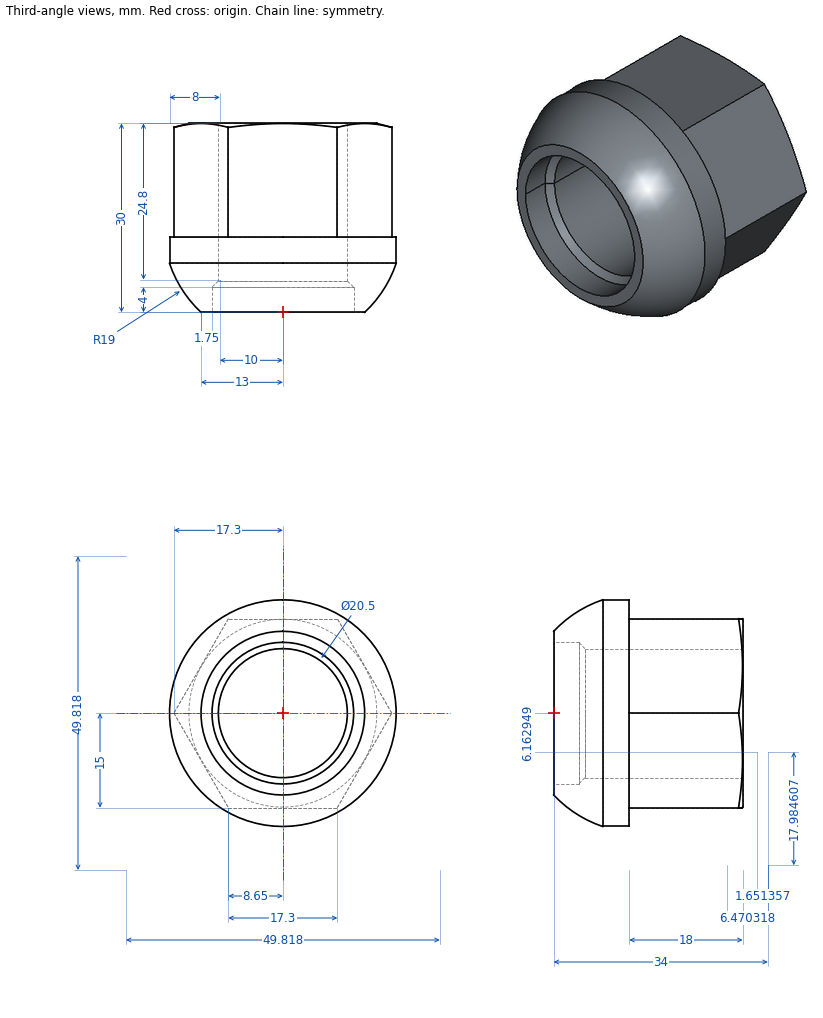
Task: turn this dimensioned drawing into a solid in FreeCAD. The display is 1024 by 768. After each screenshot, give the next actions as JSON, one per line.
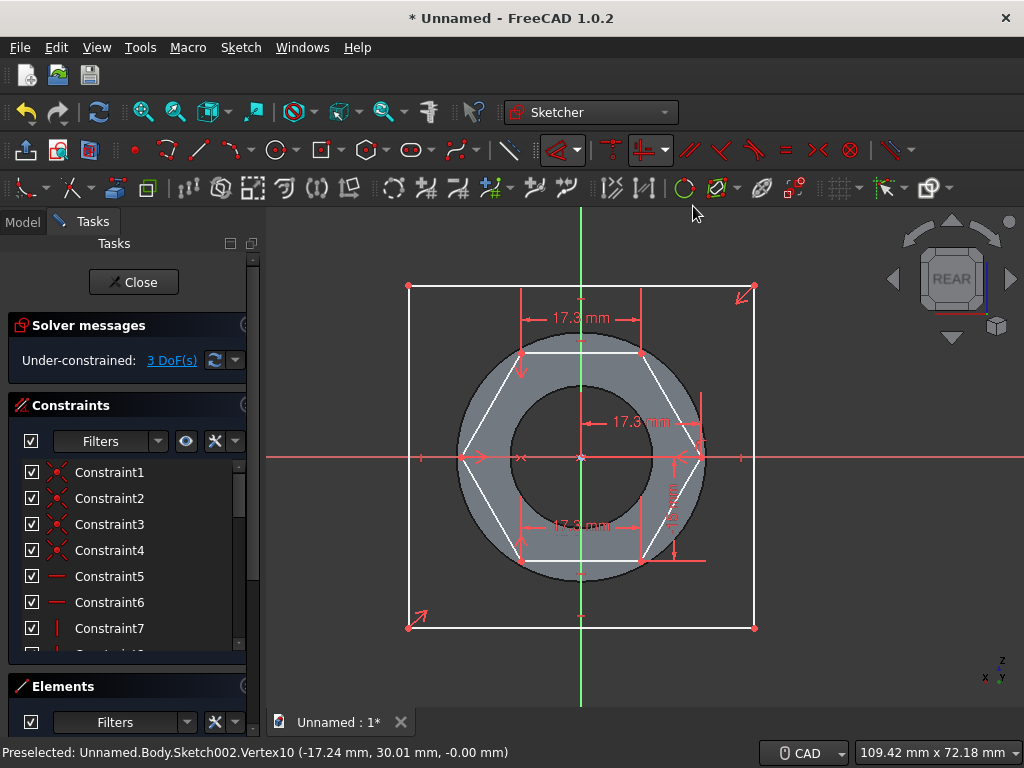
{"action": "left_click", "coordinate": [641, 561]}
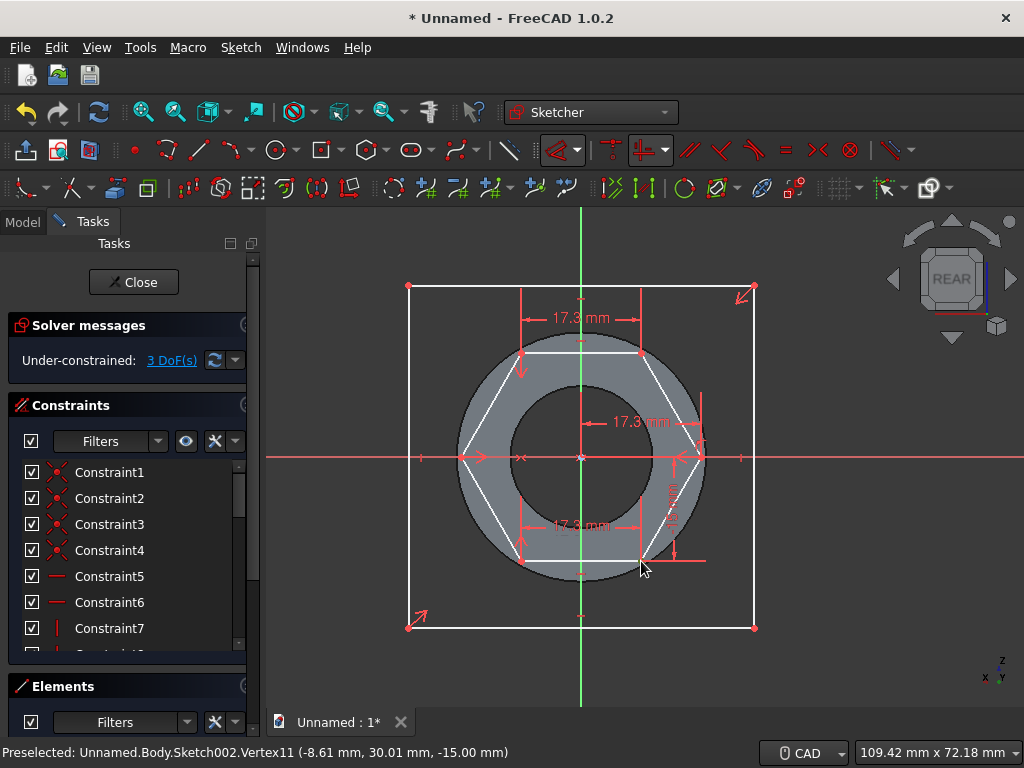
{"action": "key", "text": "l"}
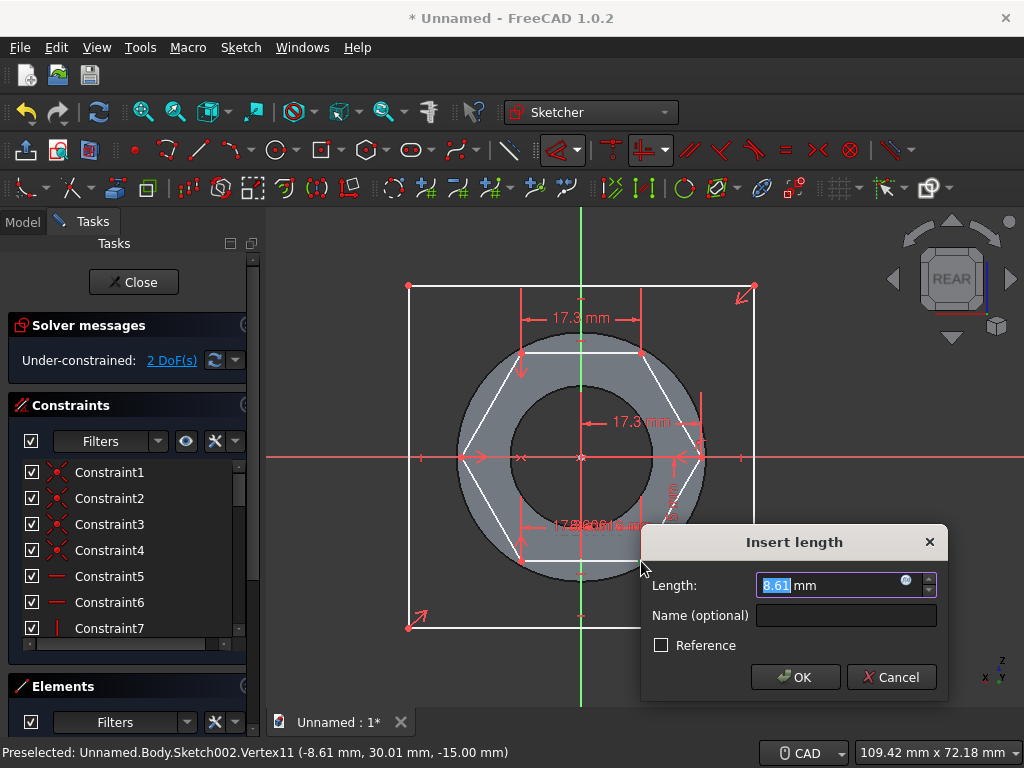
{"action": "type", "text": "8.65"}
{"action": "key", "text": "Return"}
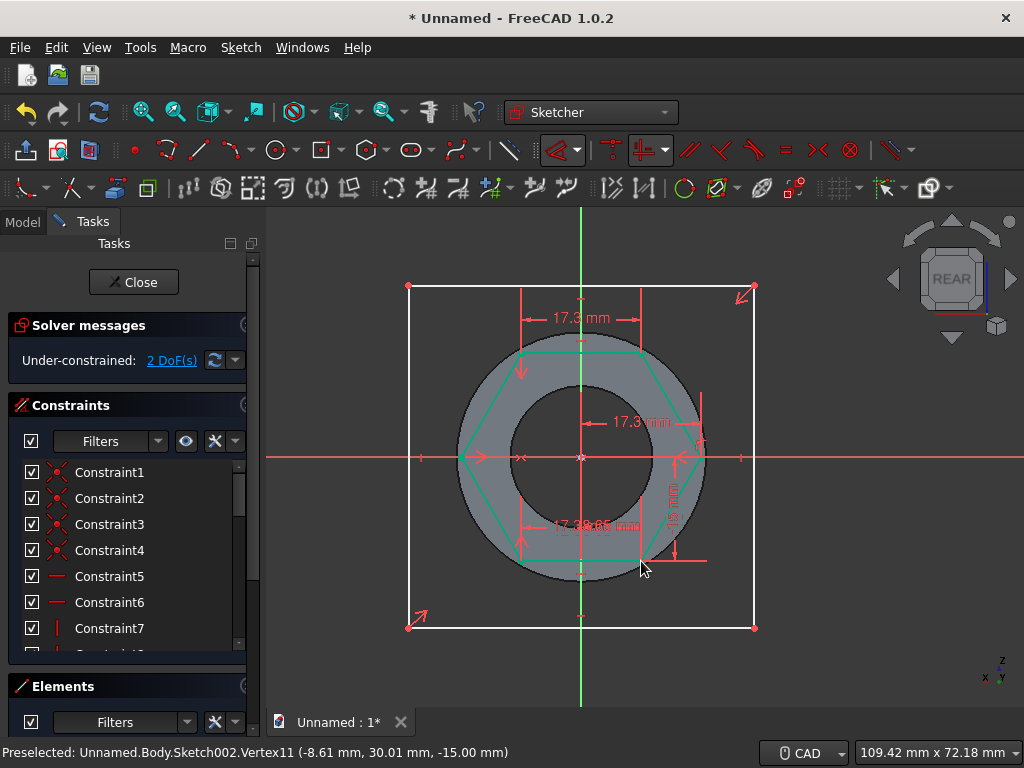
{"action": "left_click", "coordinate": [512, 628]}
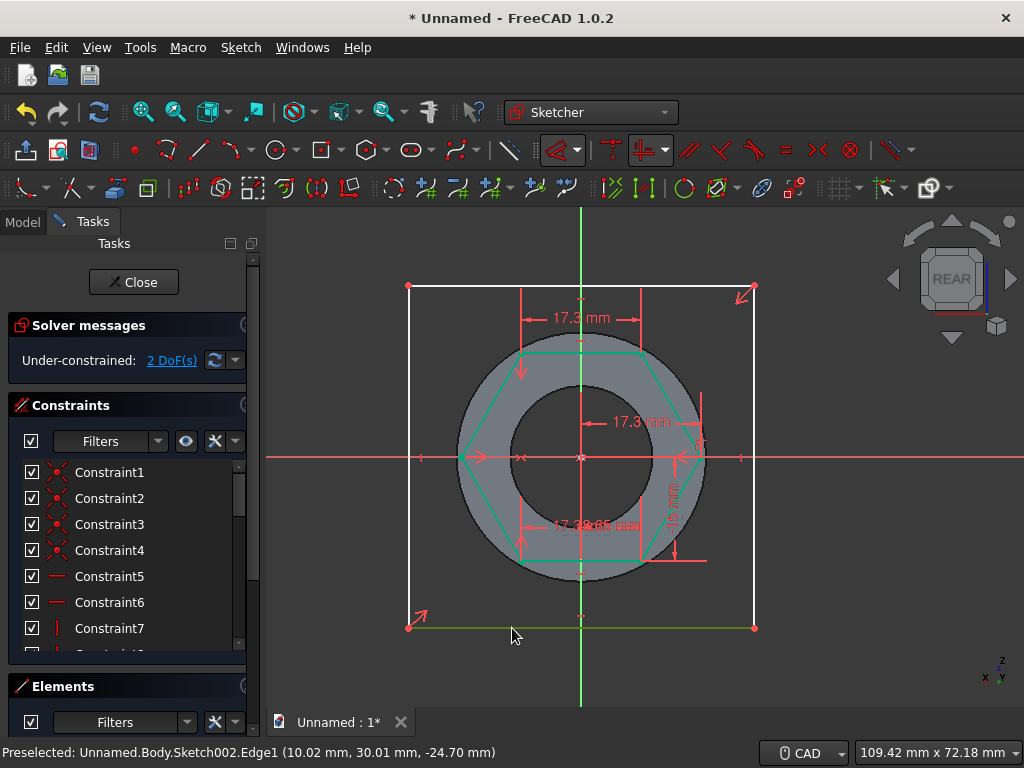
{"action": "key", "text": "l"}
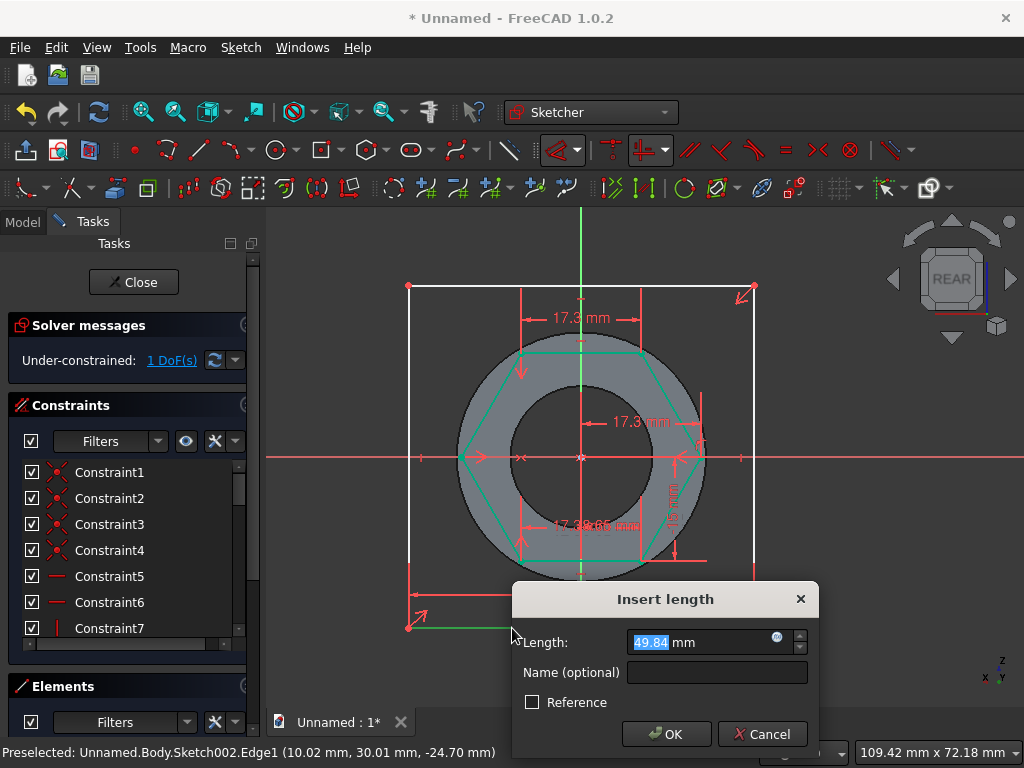
{"action": "type", "text": "49.818"}
{"action": "key", "text": "Return"}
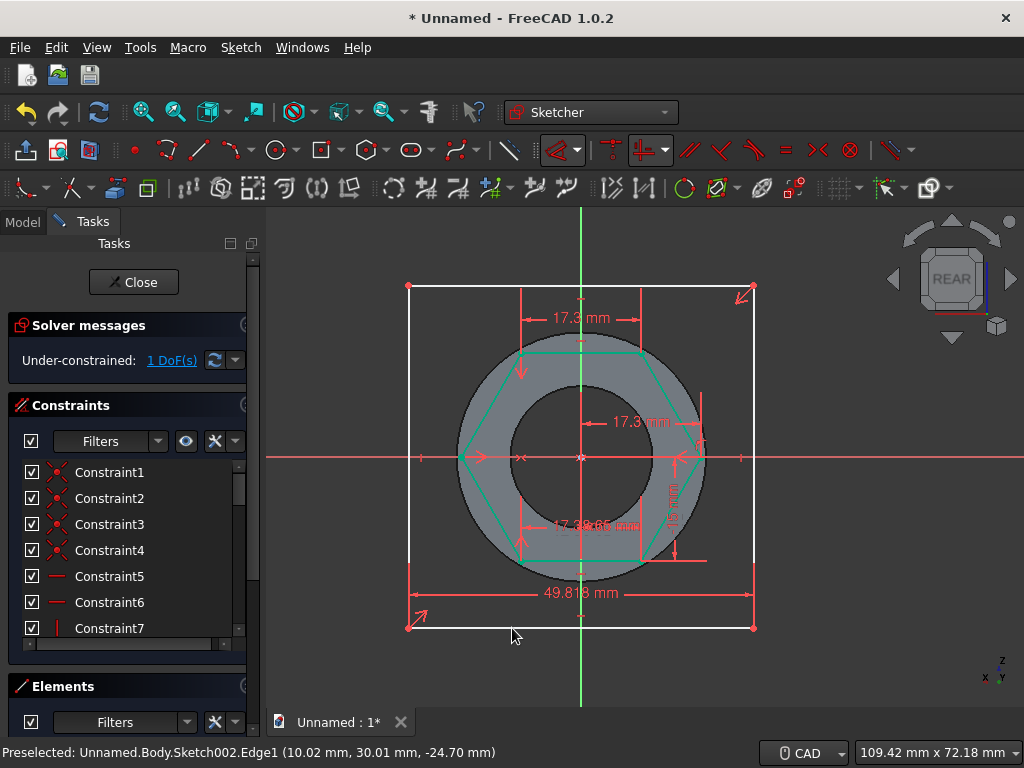
{"action": "left_click", "coordinate": [754, 526]}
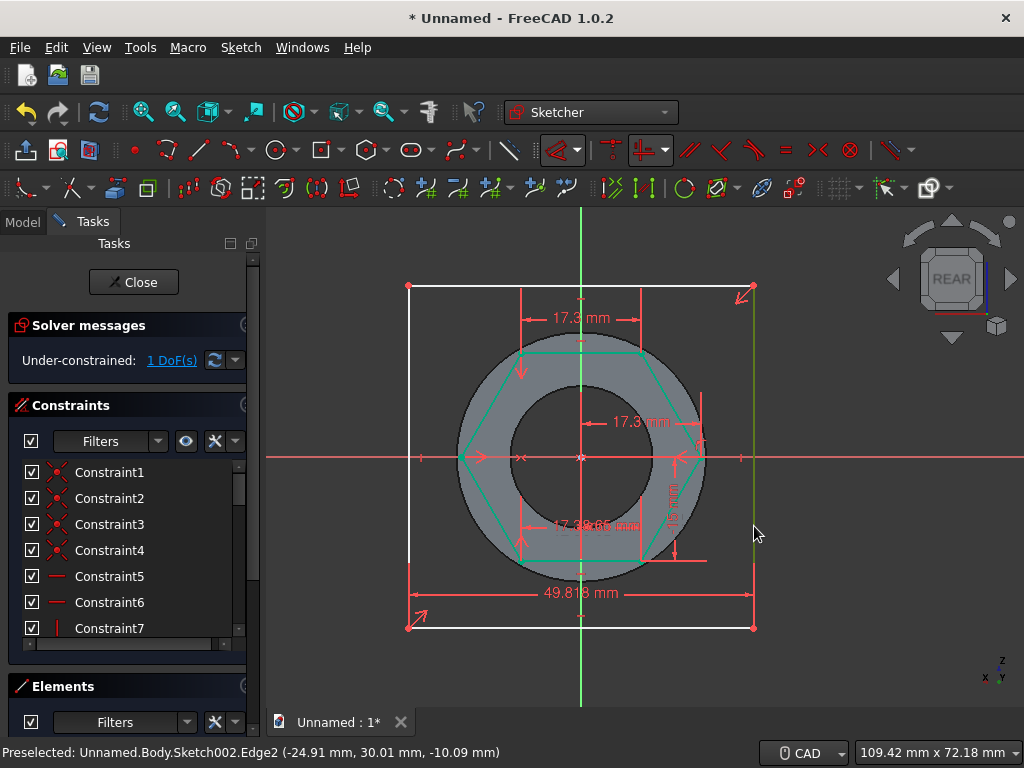
{"action": "key", "text": "i"}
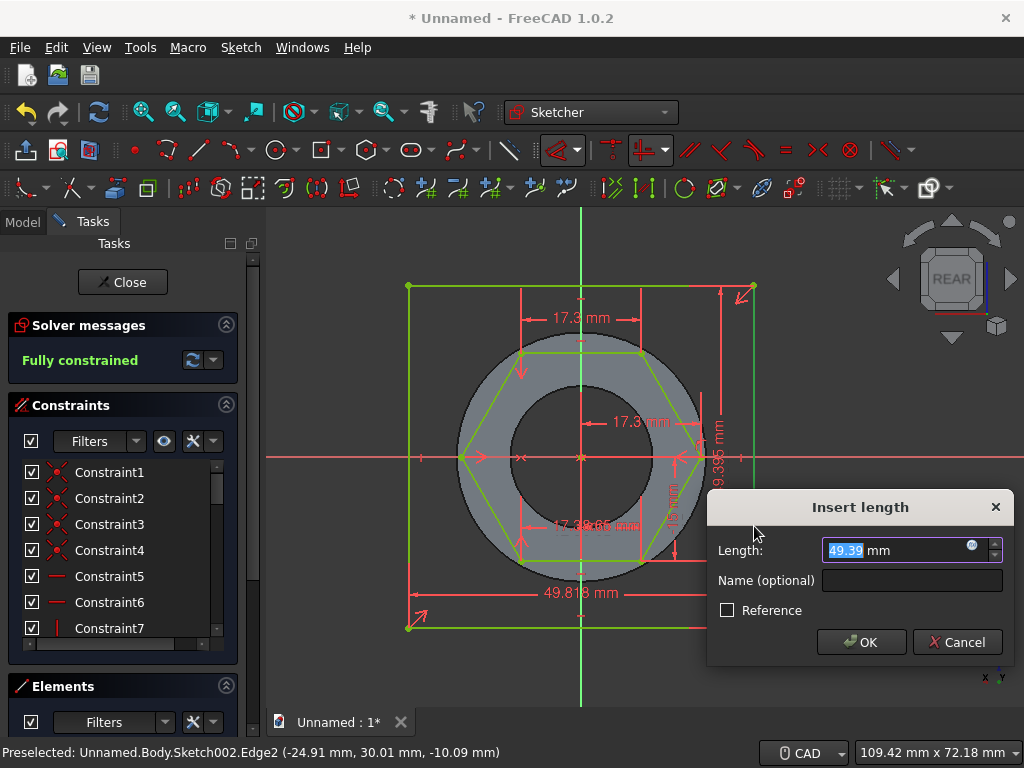
{"action": "type", "text": "49.818"}
{"action": "key", "text": "Return"}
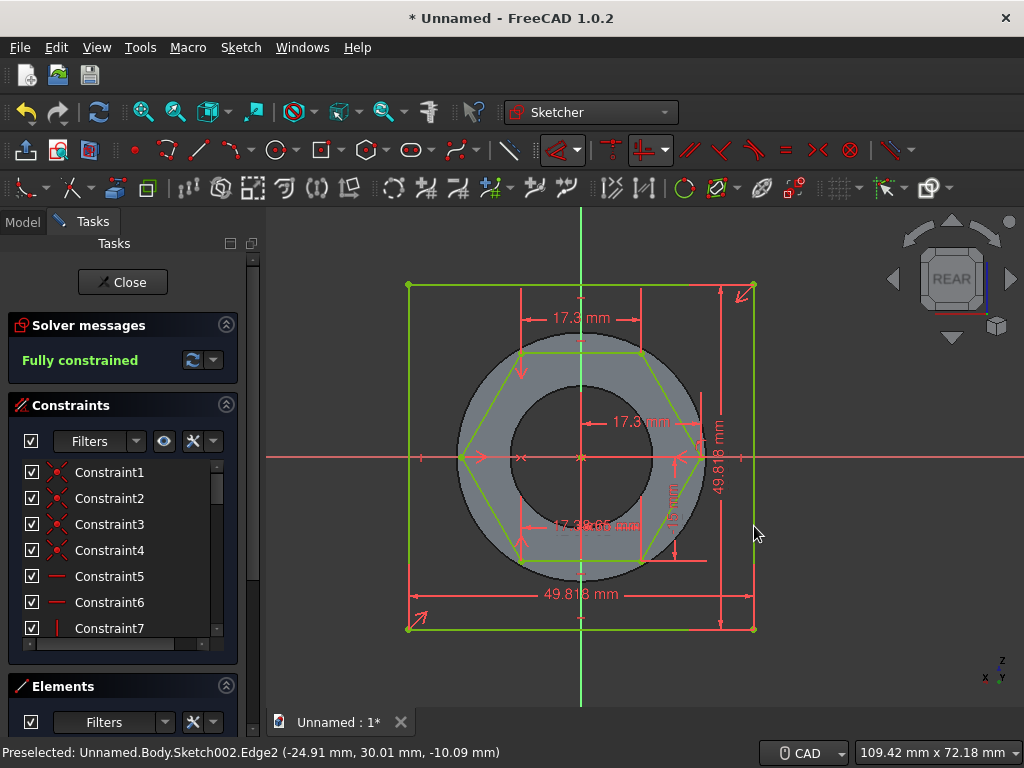
{"action": "left_click", "coordinate": [123, 282]}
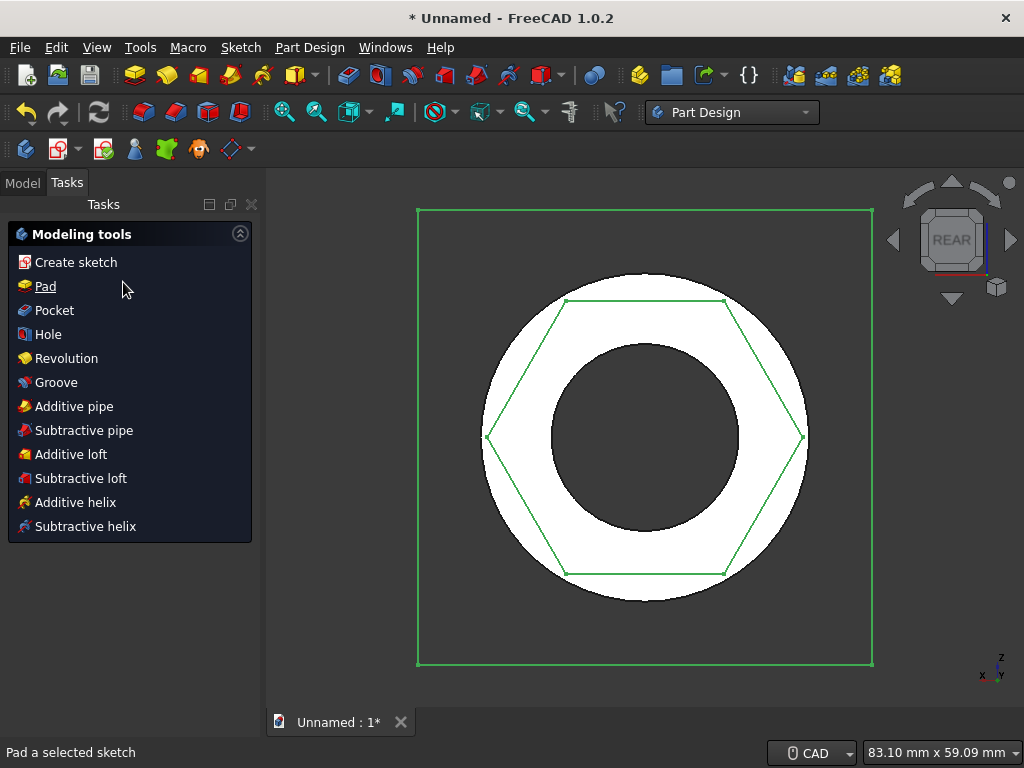
{"action": "left_click", "coordinate": [350, 76]}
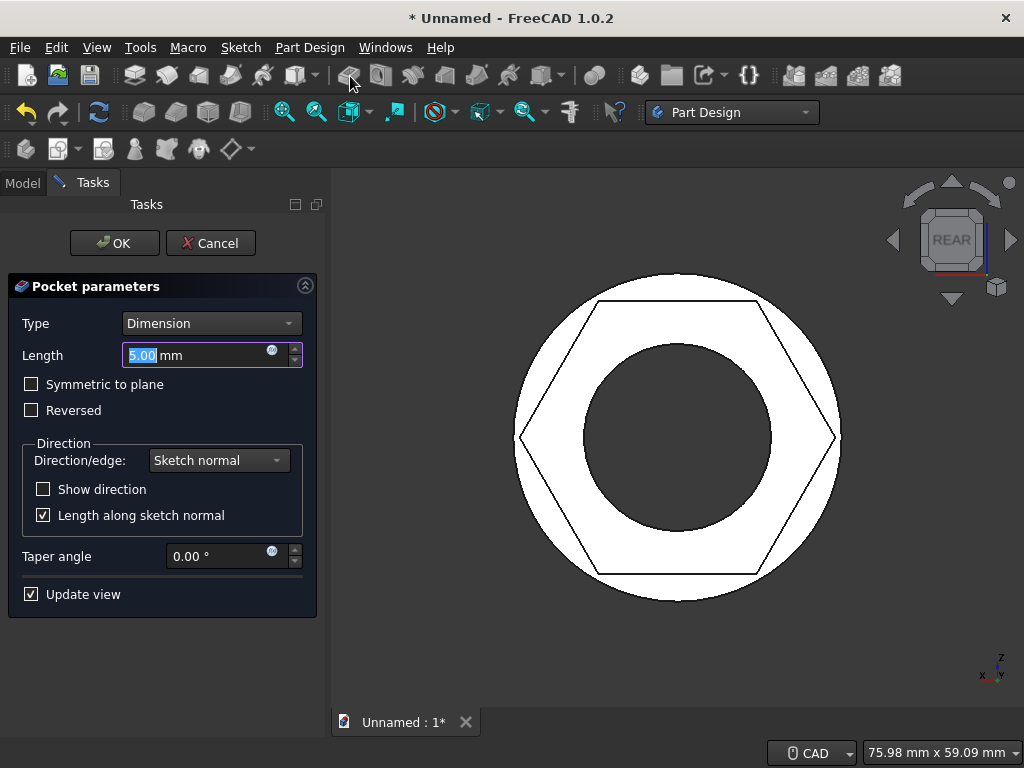
{"action": "type", "text": "18"}
{"action": "key", "text": "Tab"}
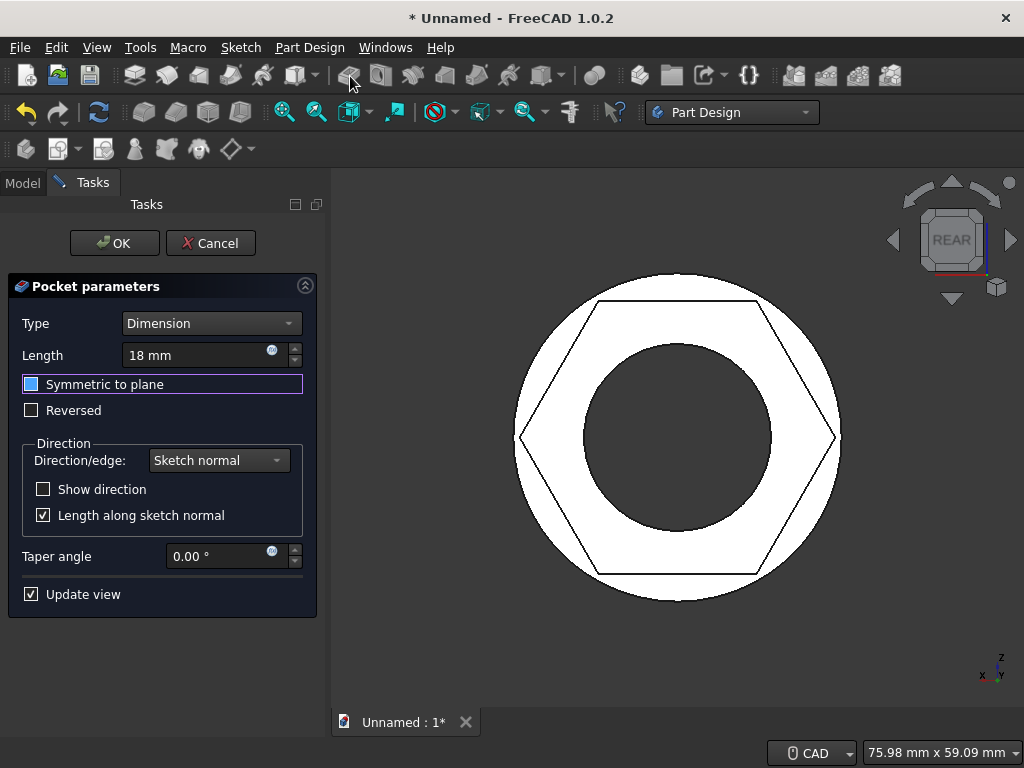
{"action": "left_click", "coordinate": [115, 243]}